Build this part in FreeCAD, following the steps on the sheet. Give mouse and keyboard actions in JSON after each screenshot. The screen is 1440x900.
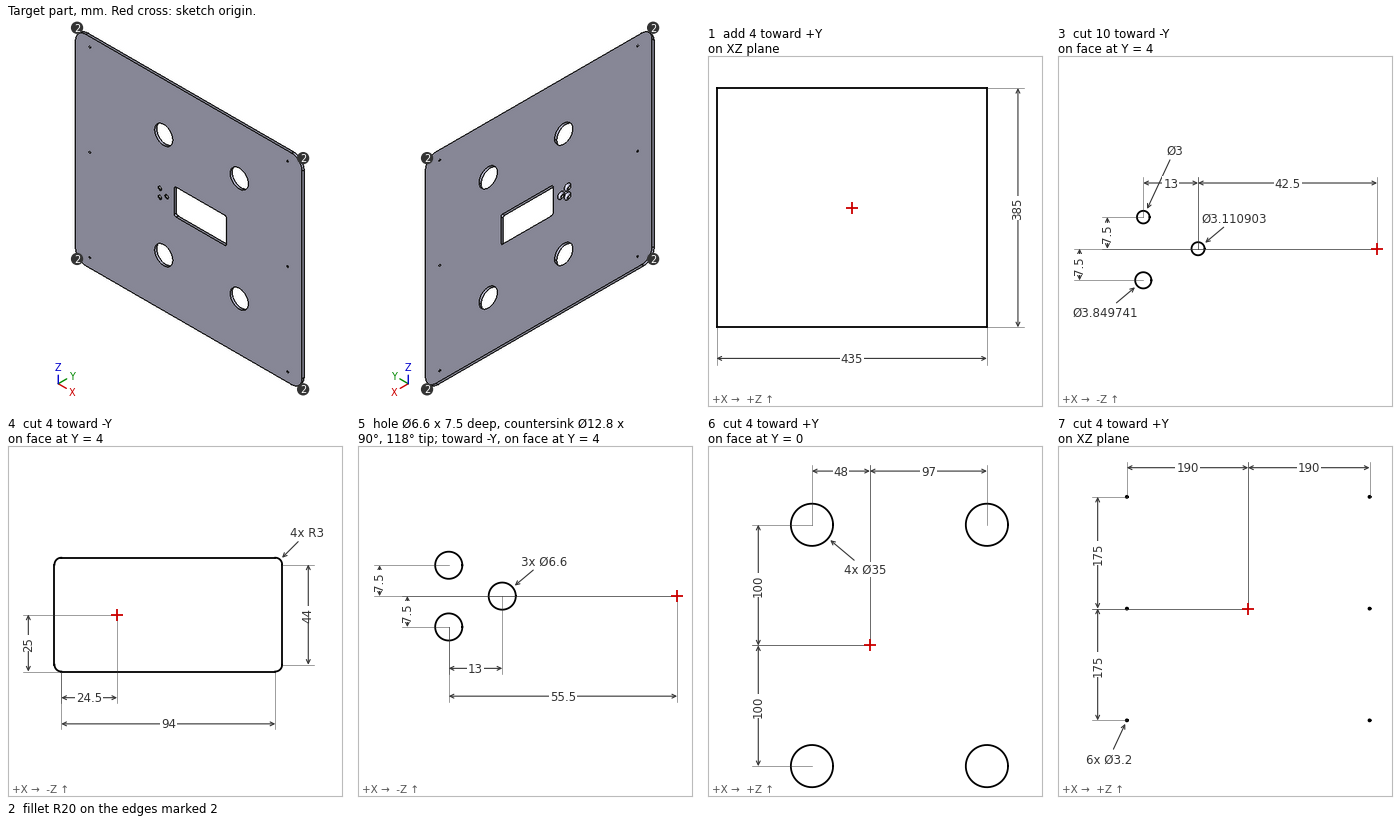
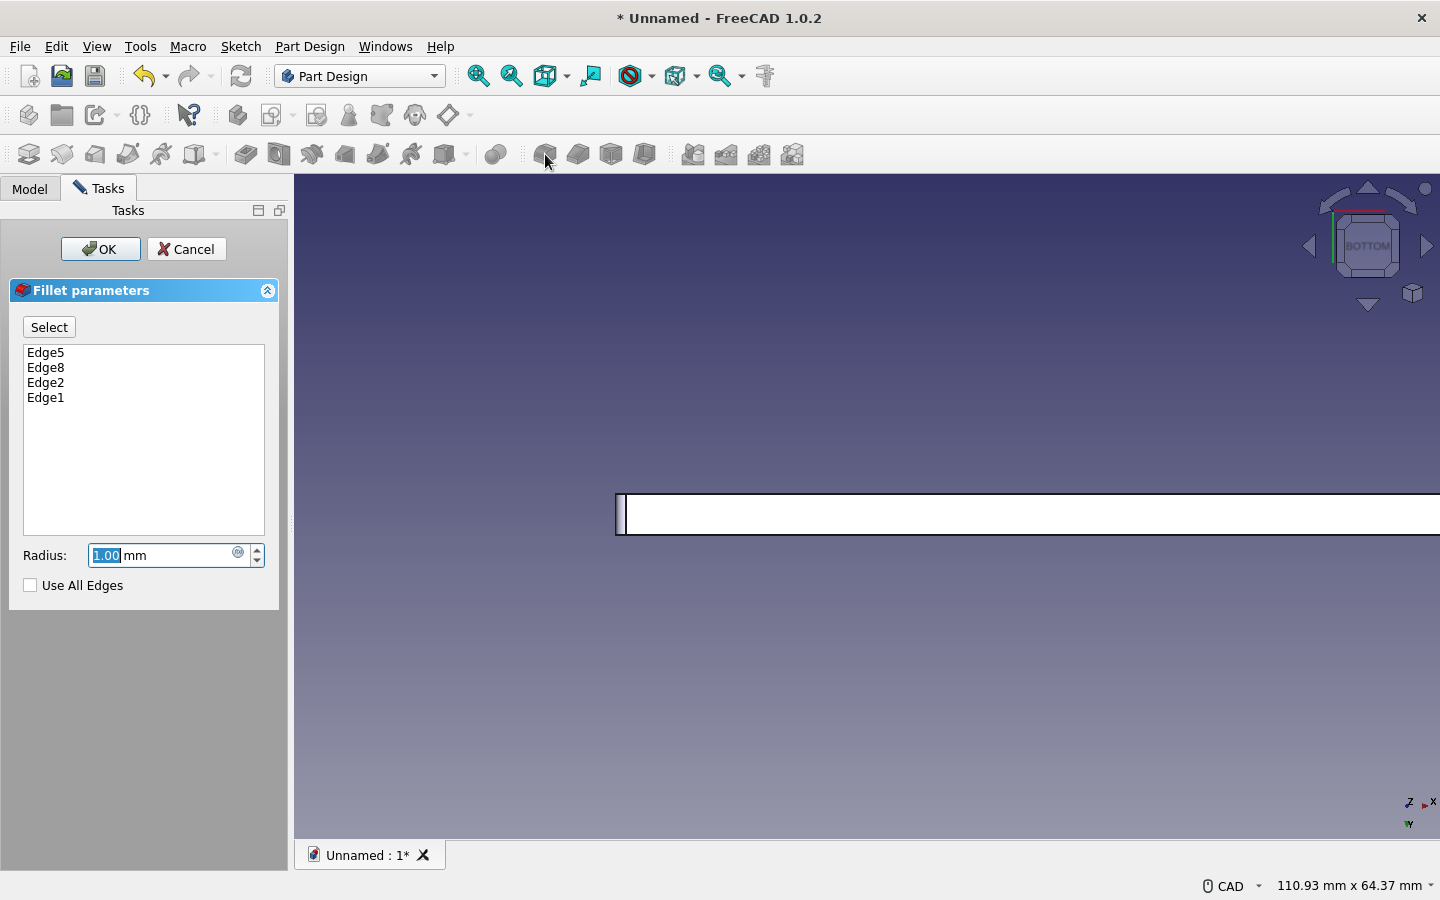
{"action": "type", "text": "20"}
{"action": "key", "text": "Tab"}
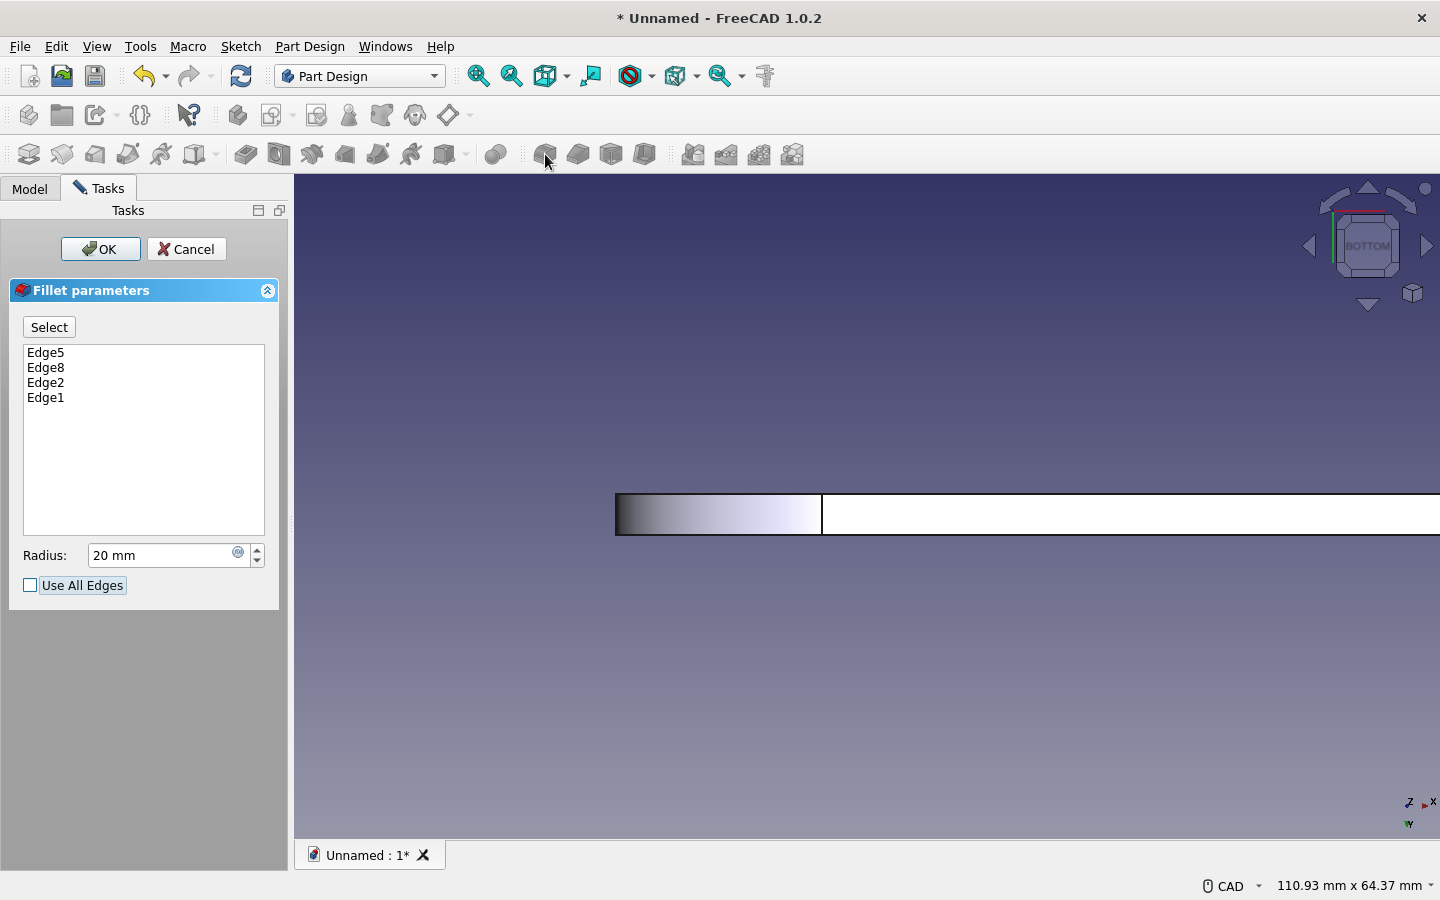
{"action": "left_click", "coordinate": [101, 249]}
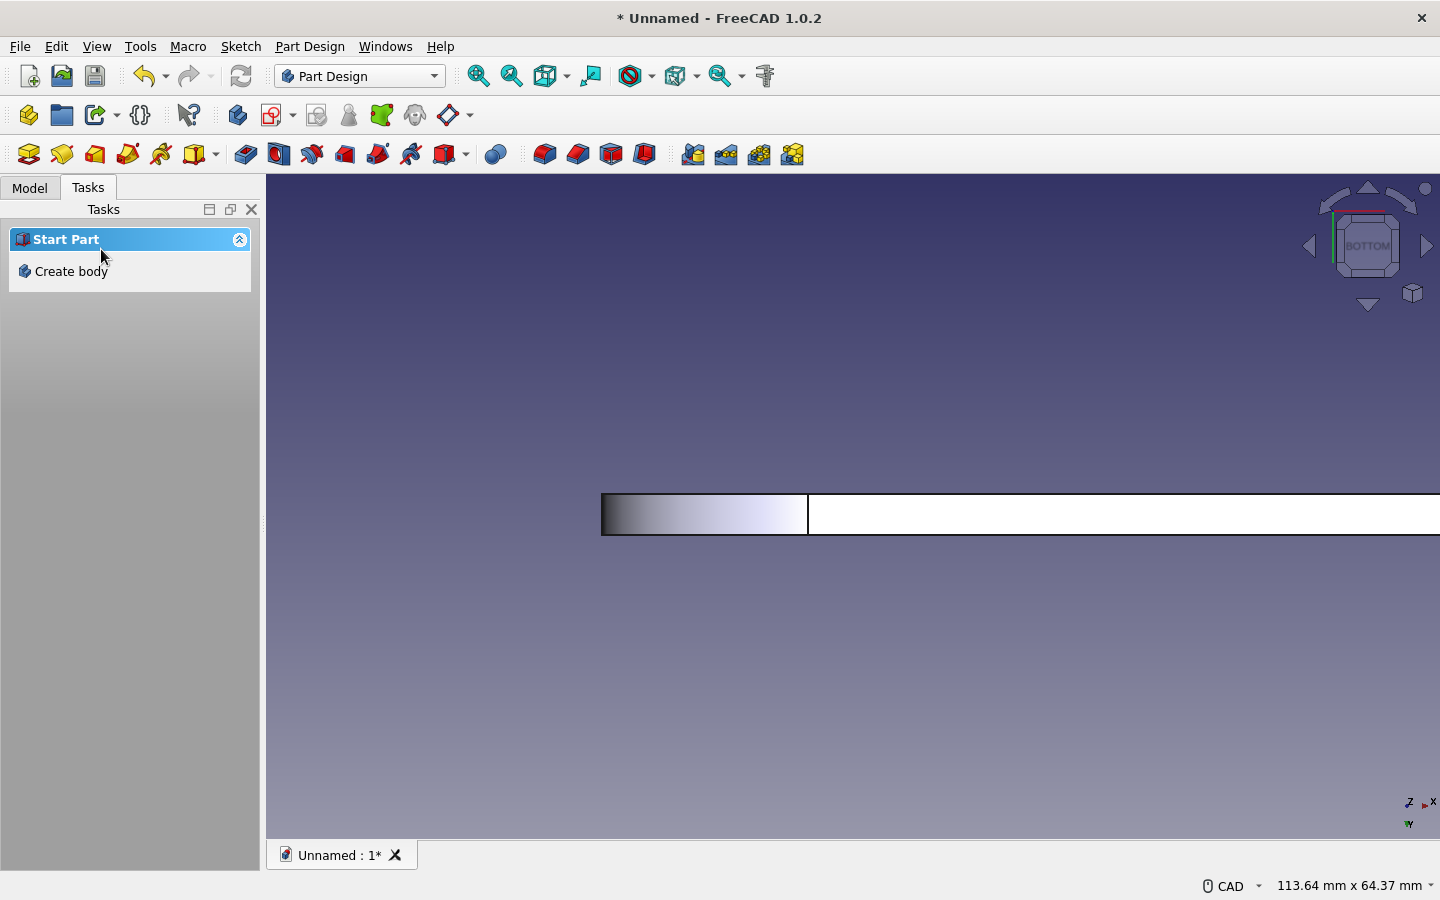
{"action": "left_click", "coordinate": [479, 76]}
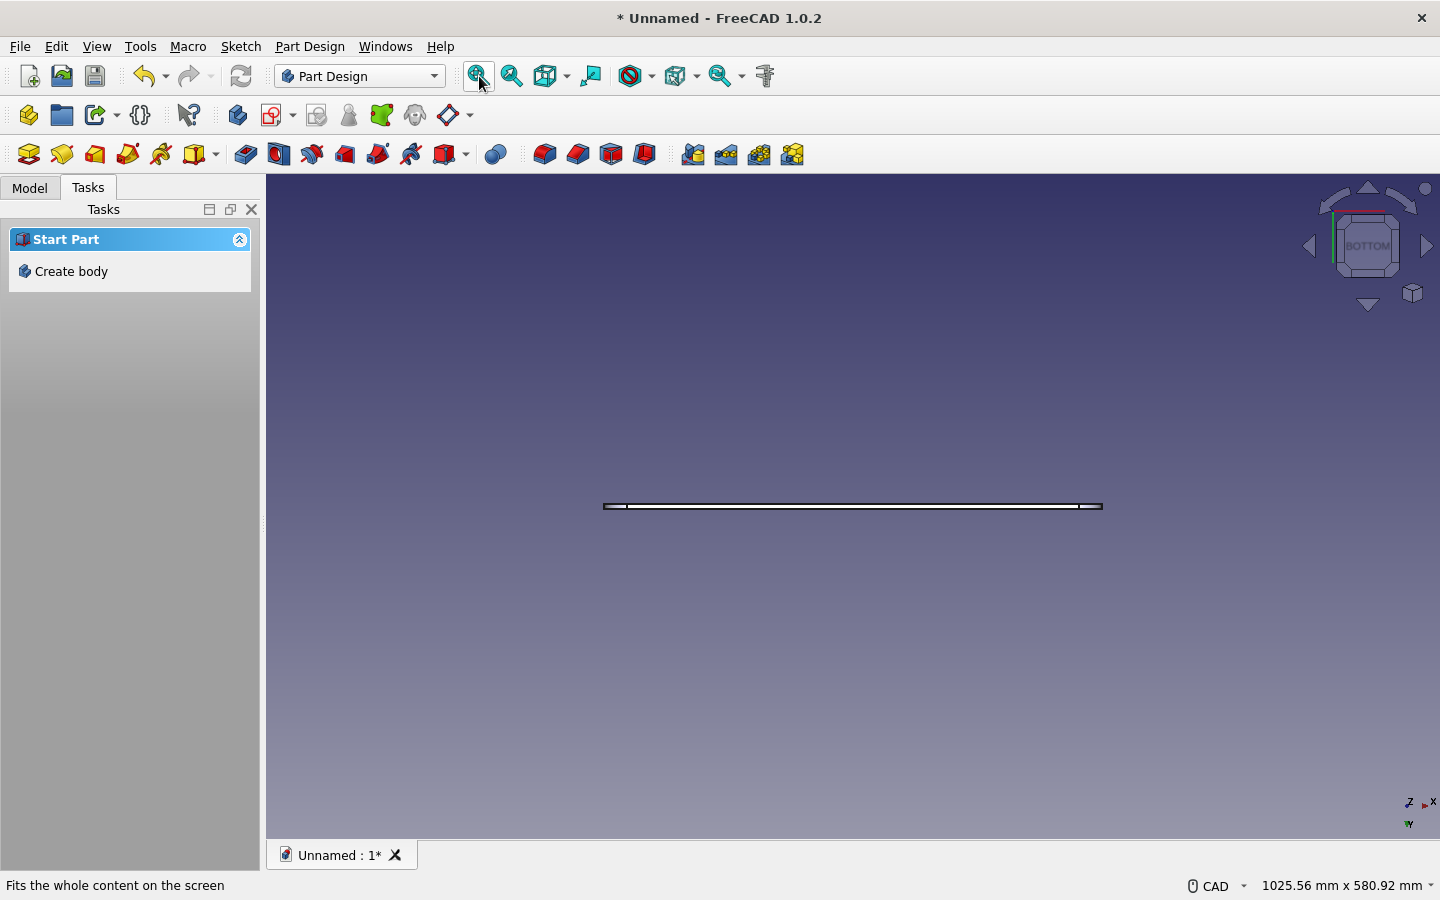
{"action": "key", "text": "4"}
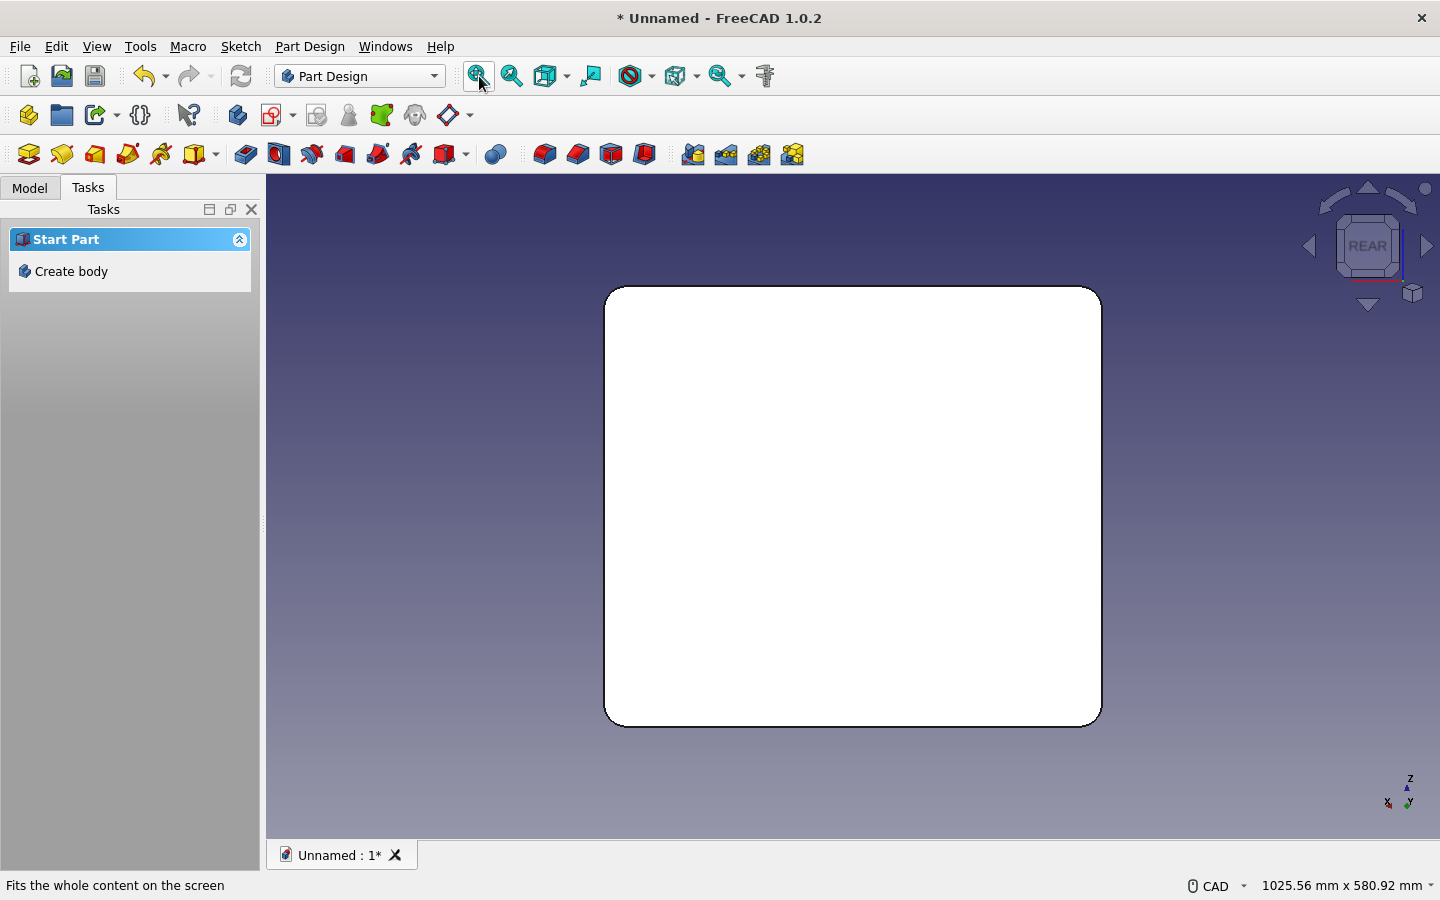
{"action": "left_click", "coordinate": [853, 505]}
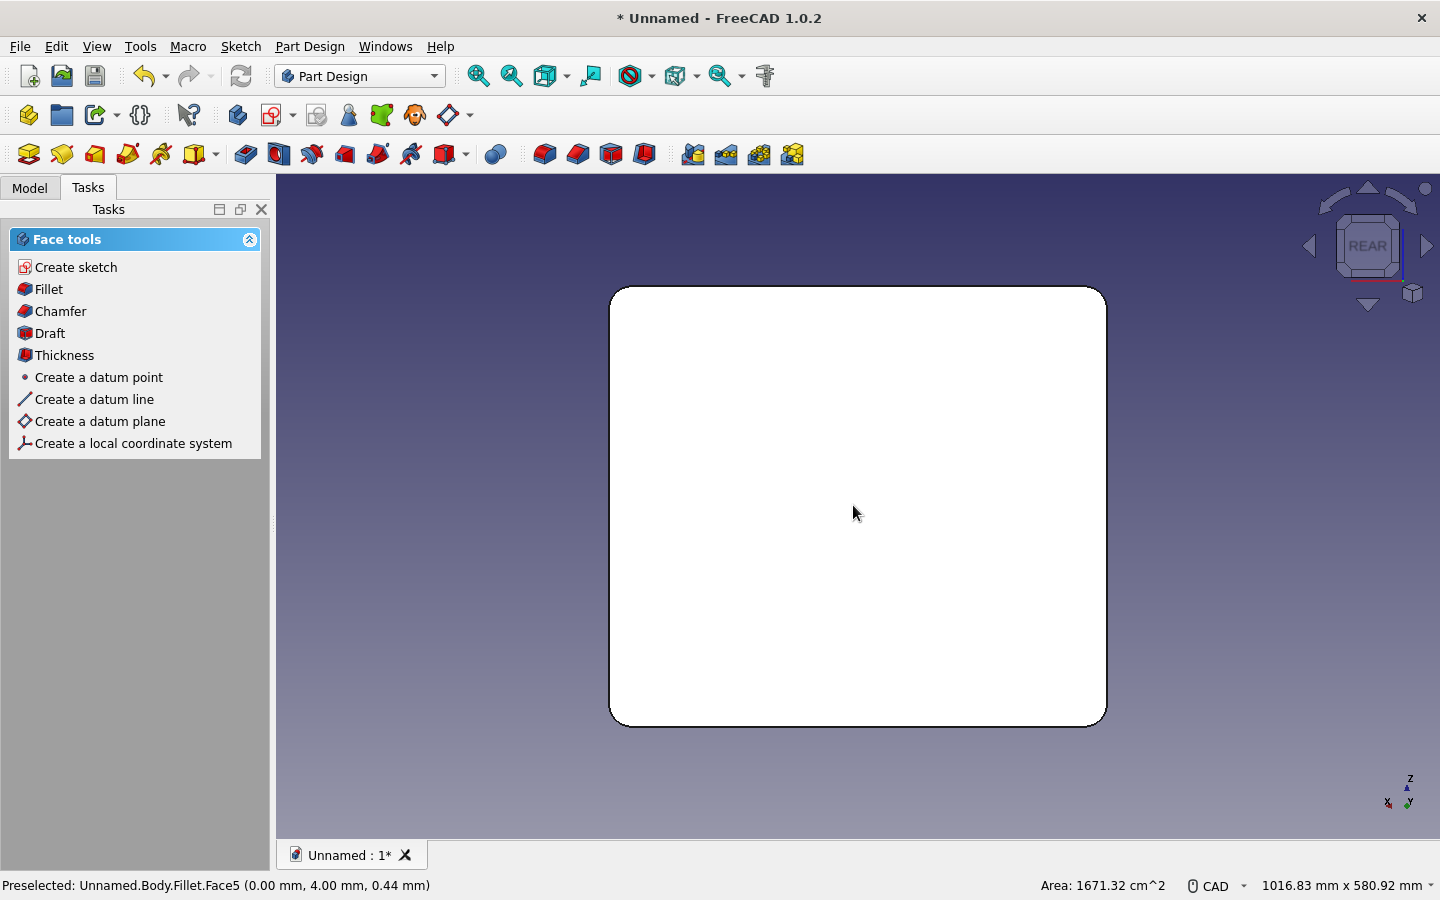
{"action": "left_click", "coordinate": [270, 116]}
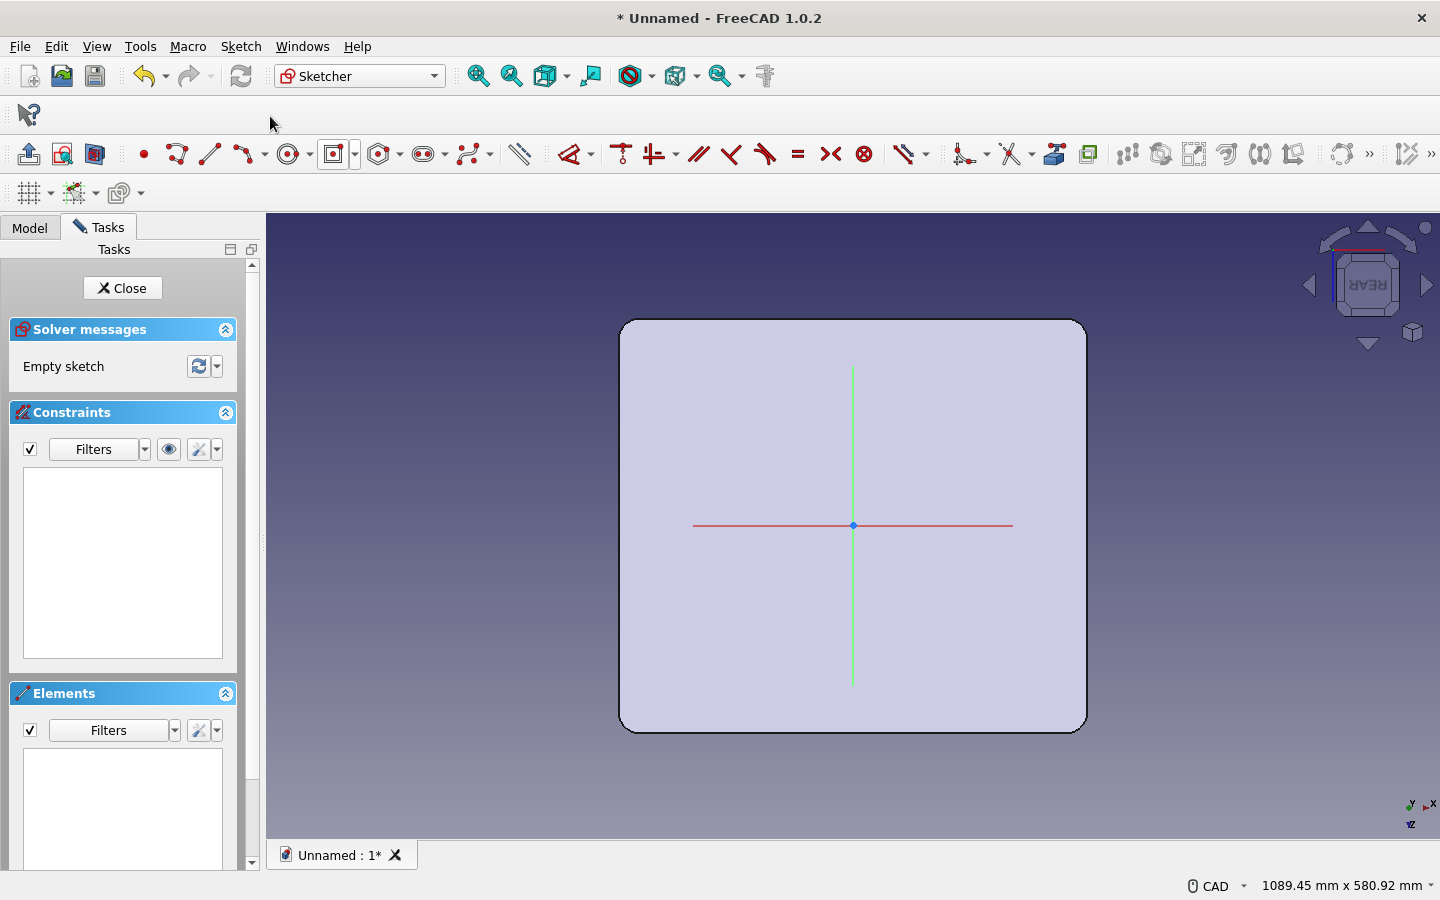
{"action": "scroll", "coordinate": [801, 526], "scroll_direction": "up", "scroll_amount": 15}